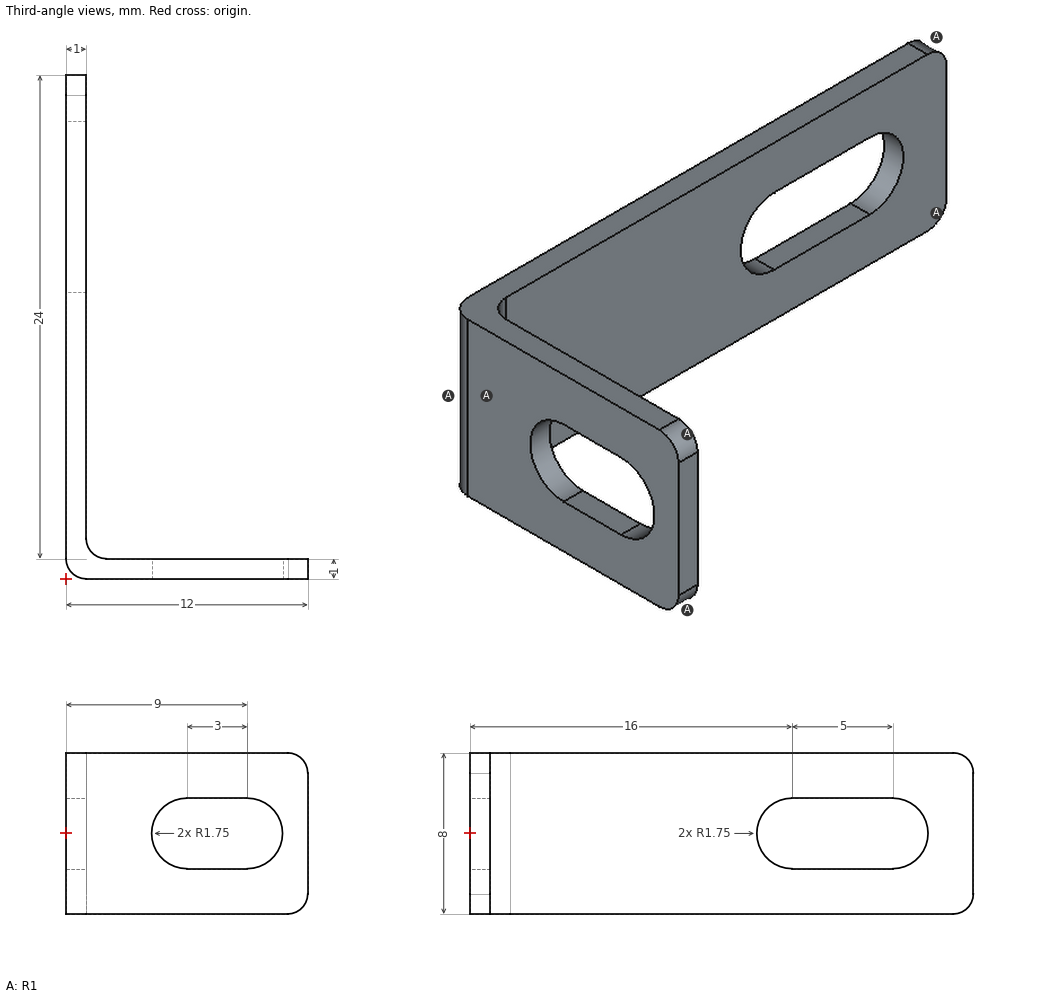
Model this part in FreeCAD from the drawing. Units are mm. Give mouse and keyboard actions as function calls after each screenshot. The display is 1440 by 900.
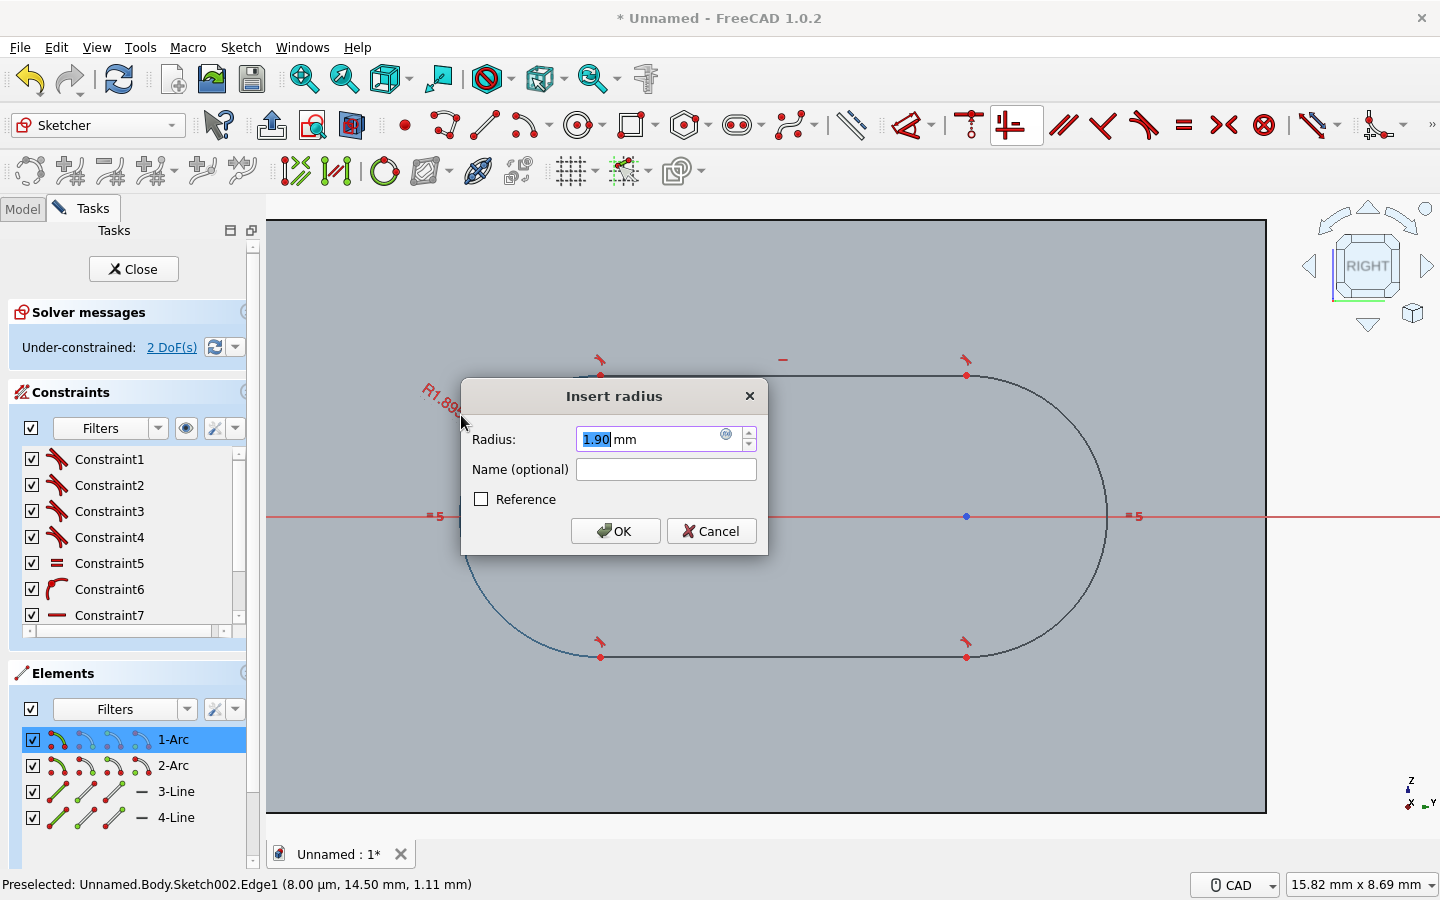
text(1.75)
key(Return)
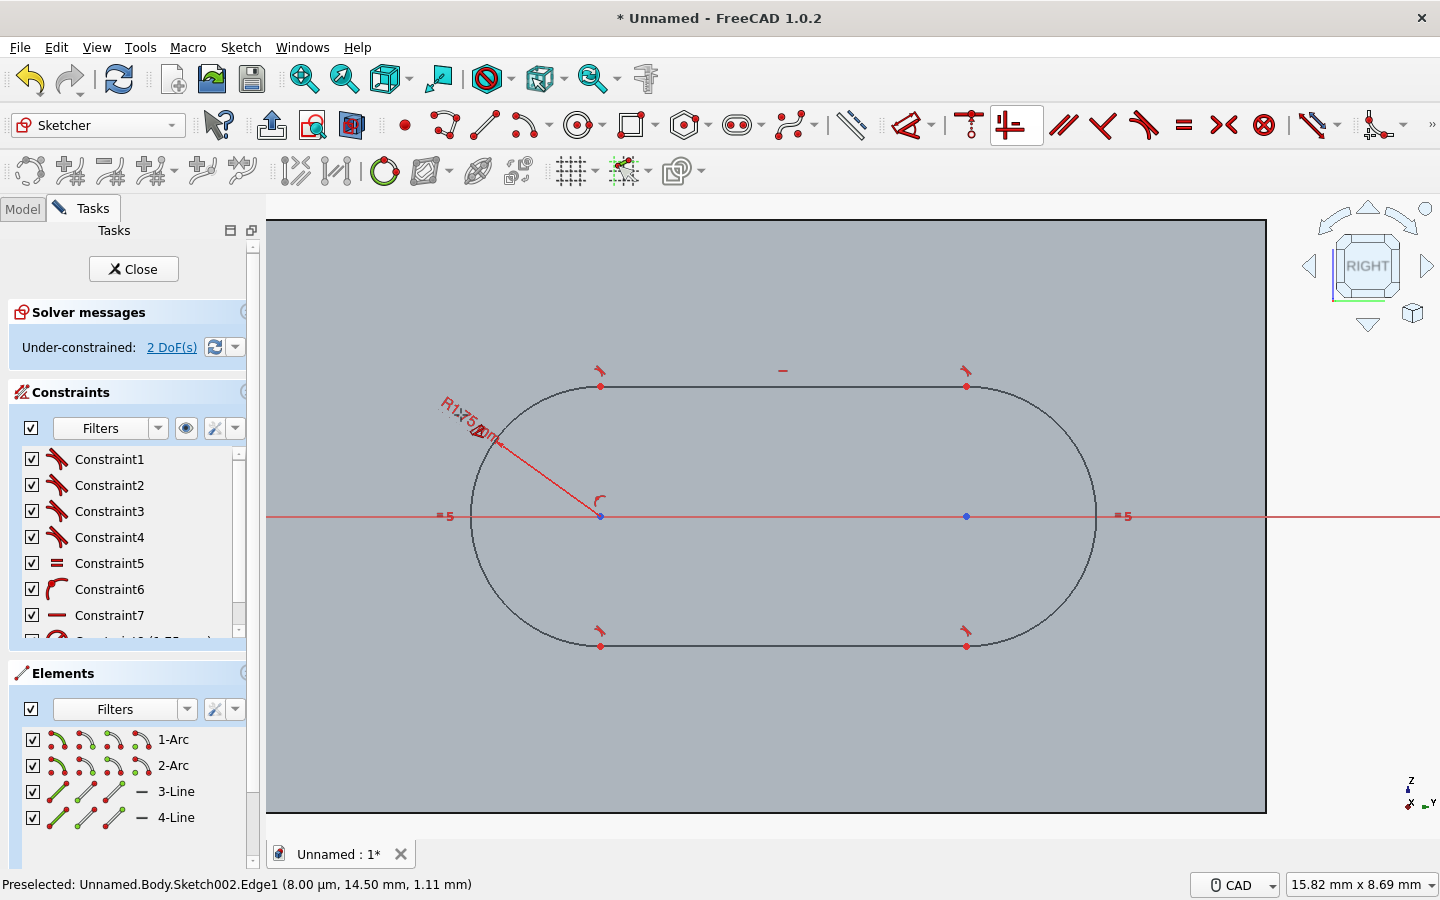
click(710, 387)
click(784, 353)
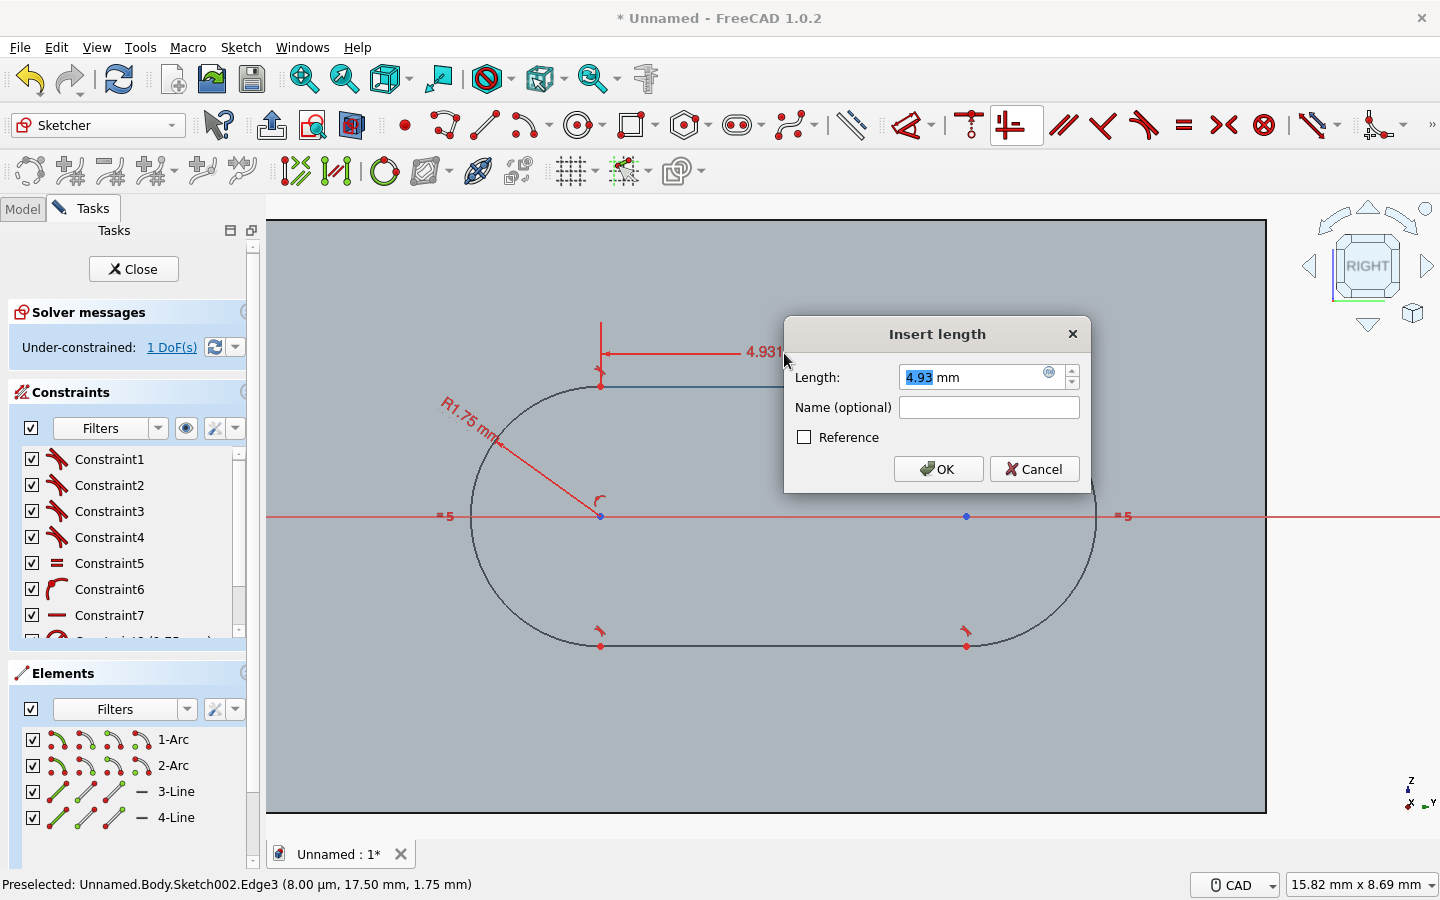
text(5)
key(Return)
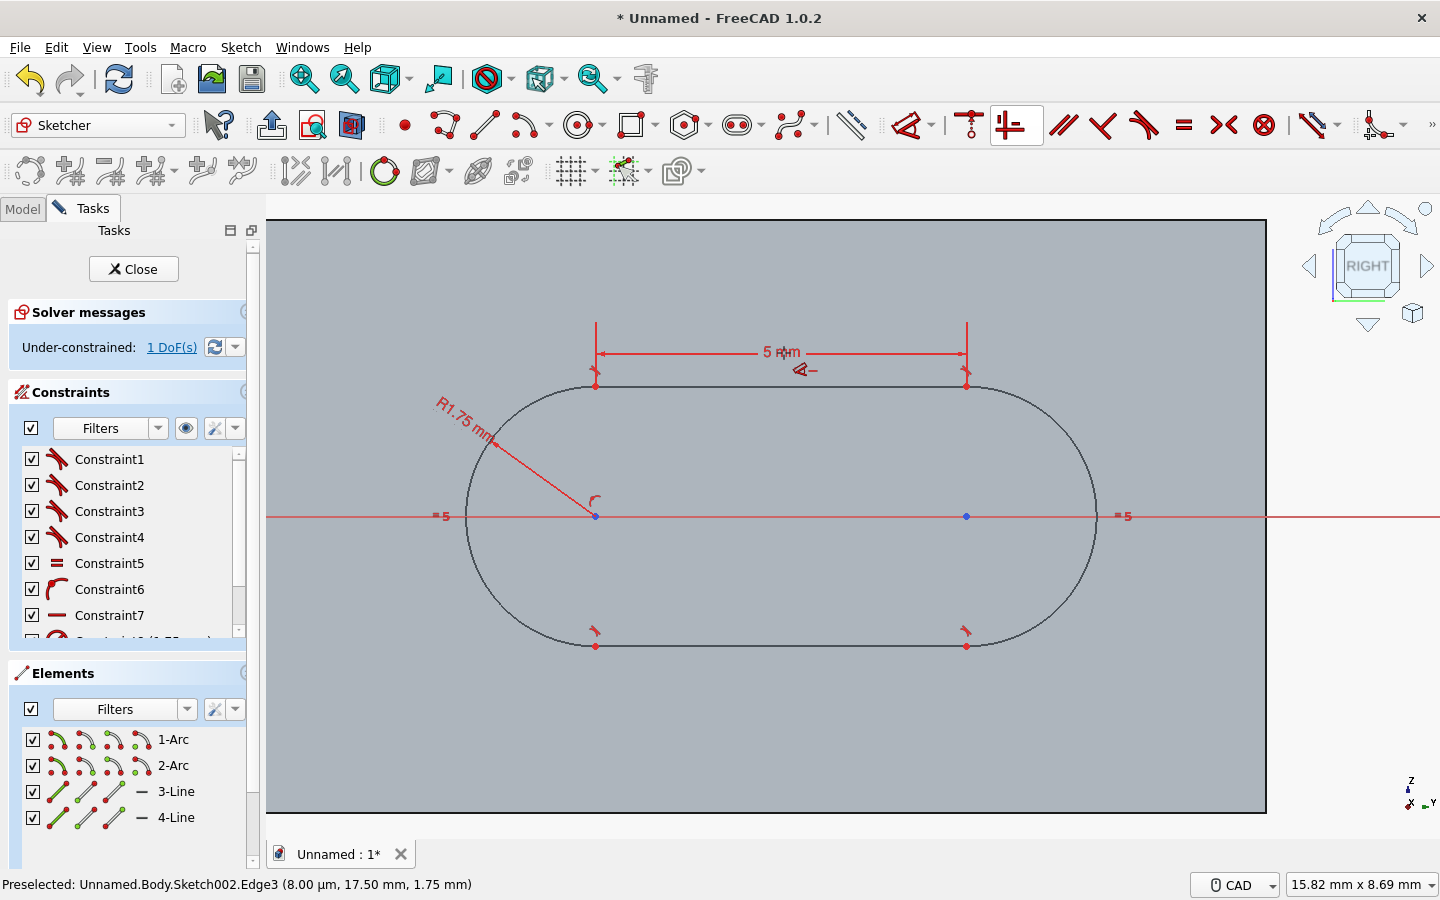
click(596, 387)
click(445, 353)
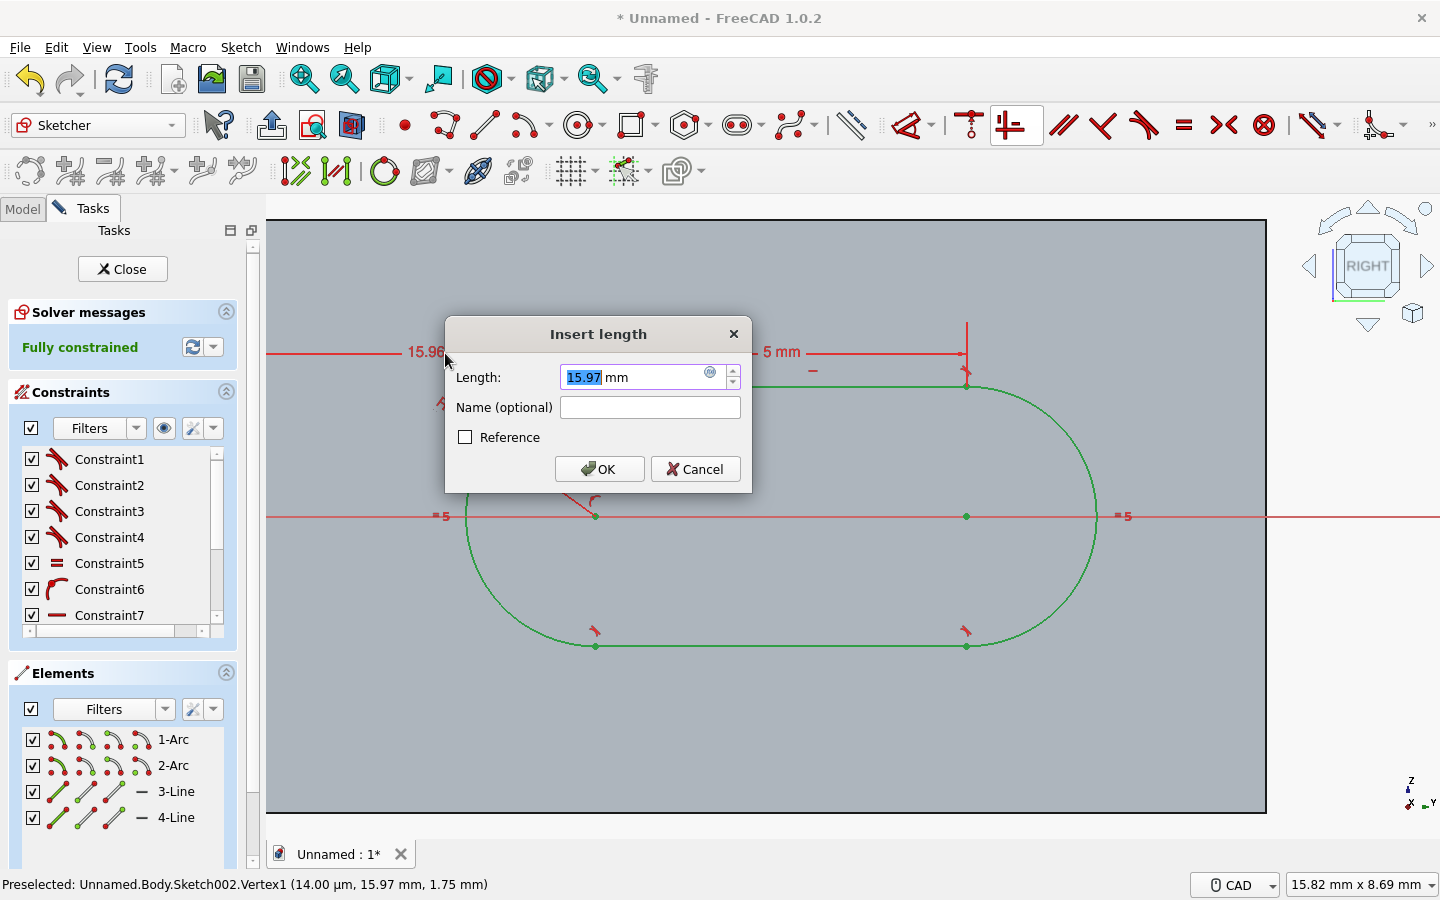
text(16)
key(Return)
key(Escape)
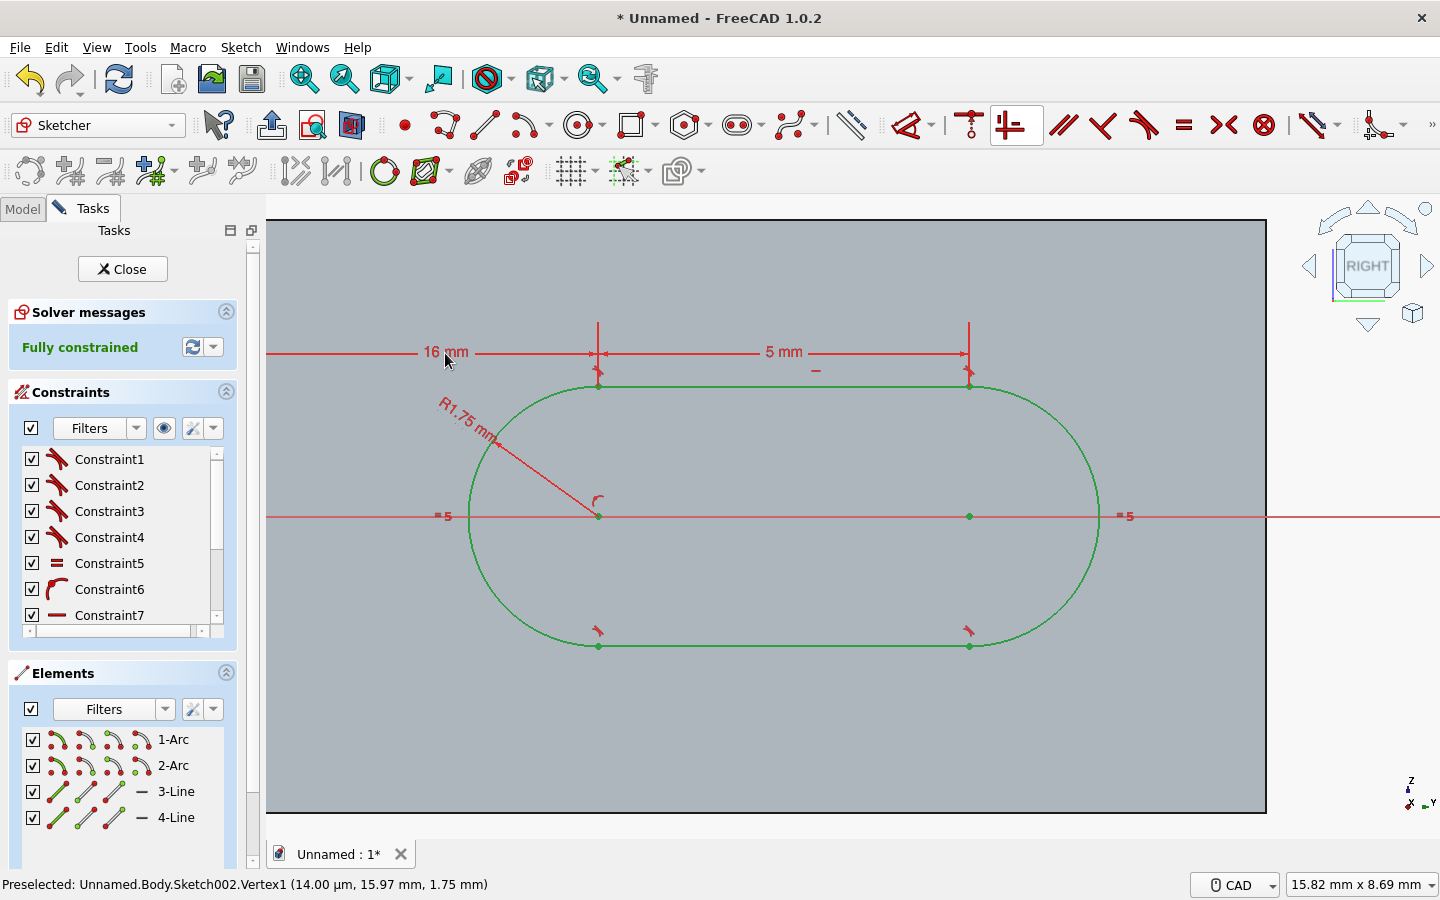
click(123, 269)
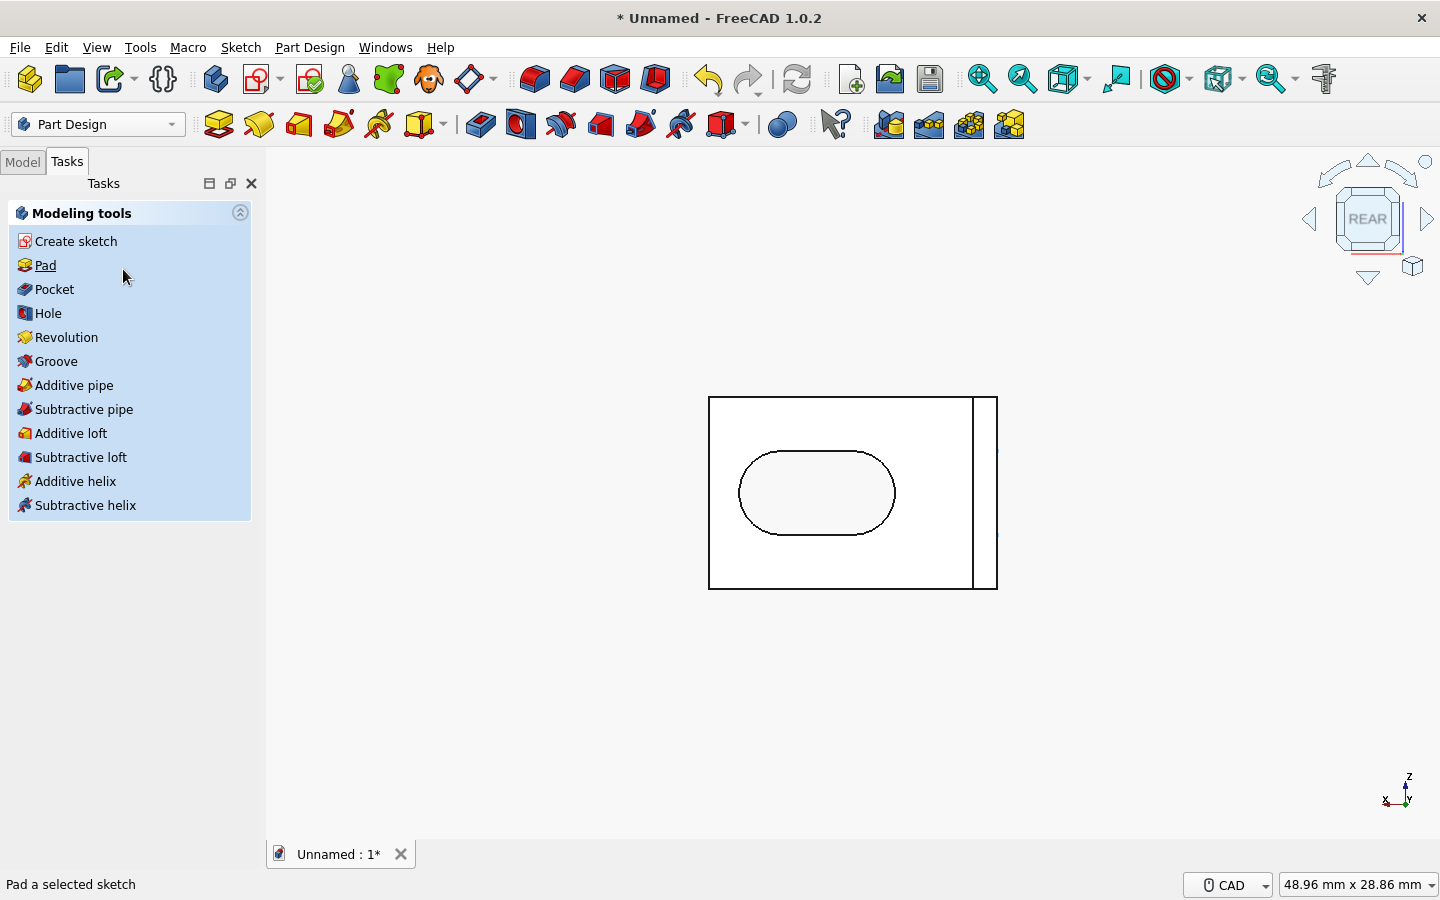
click(482, 124)